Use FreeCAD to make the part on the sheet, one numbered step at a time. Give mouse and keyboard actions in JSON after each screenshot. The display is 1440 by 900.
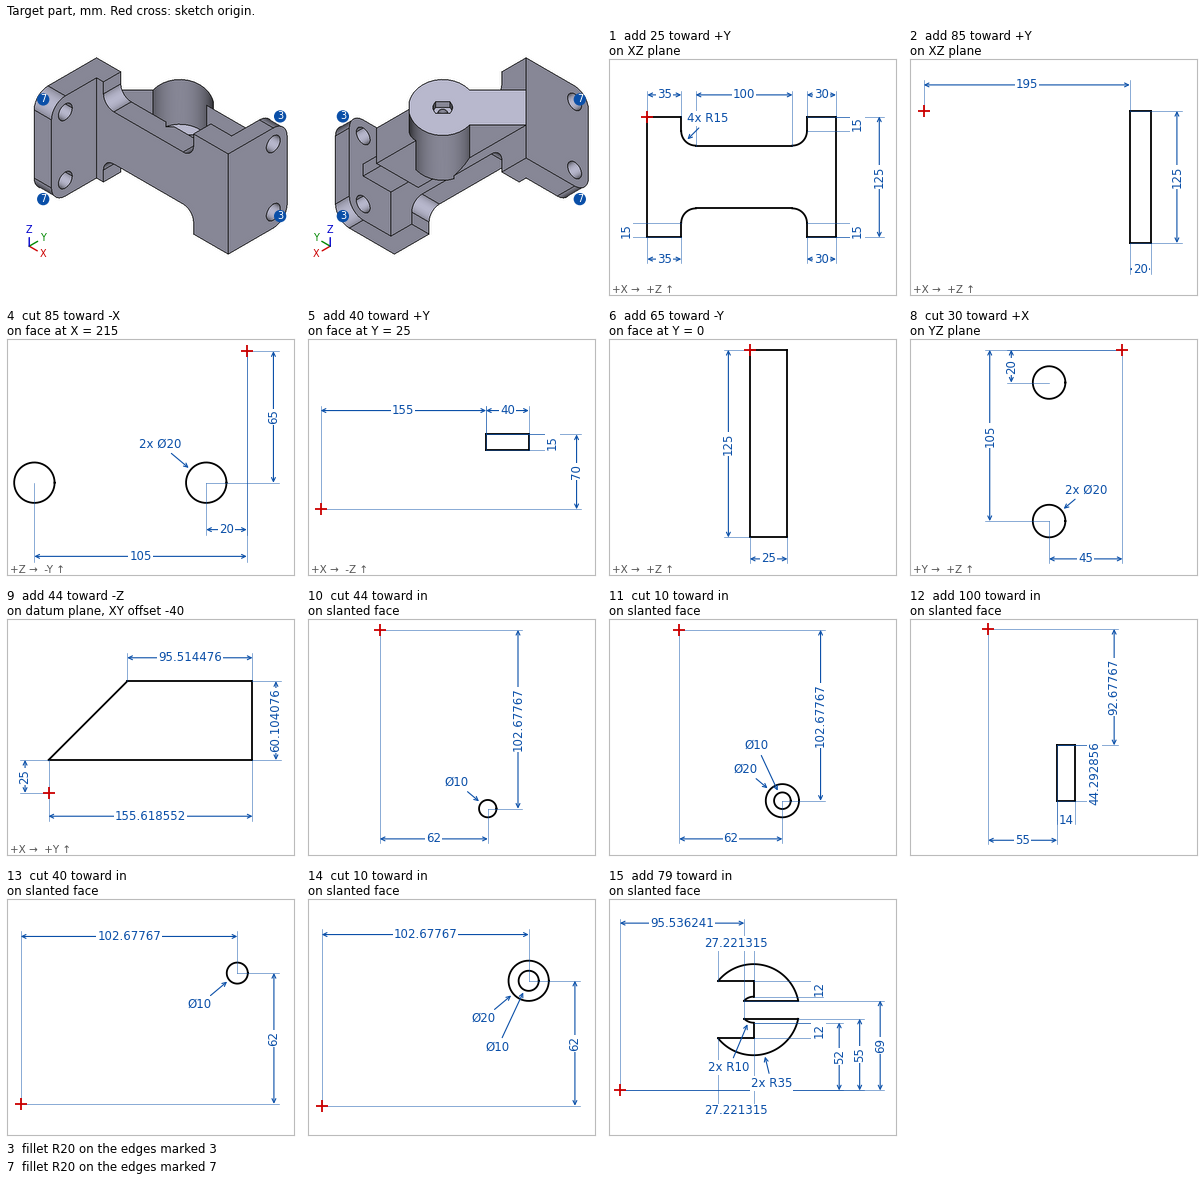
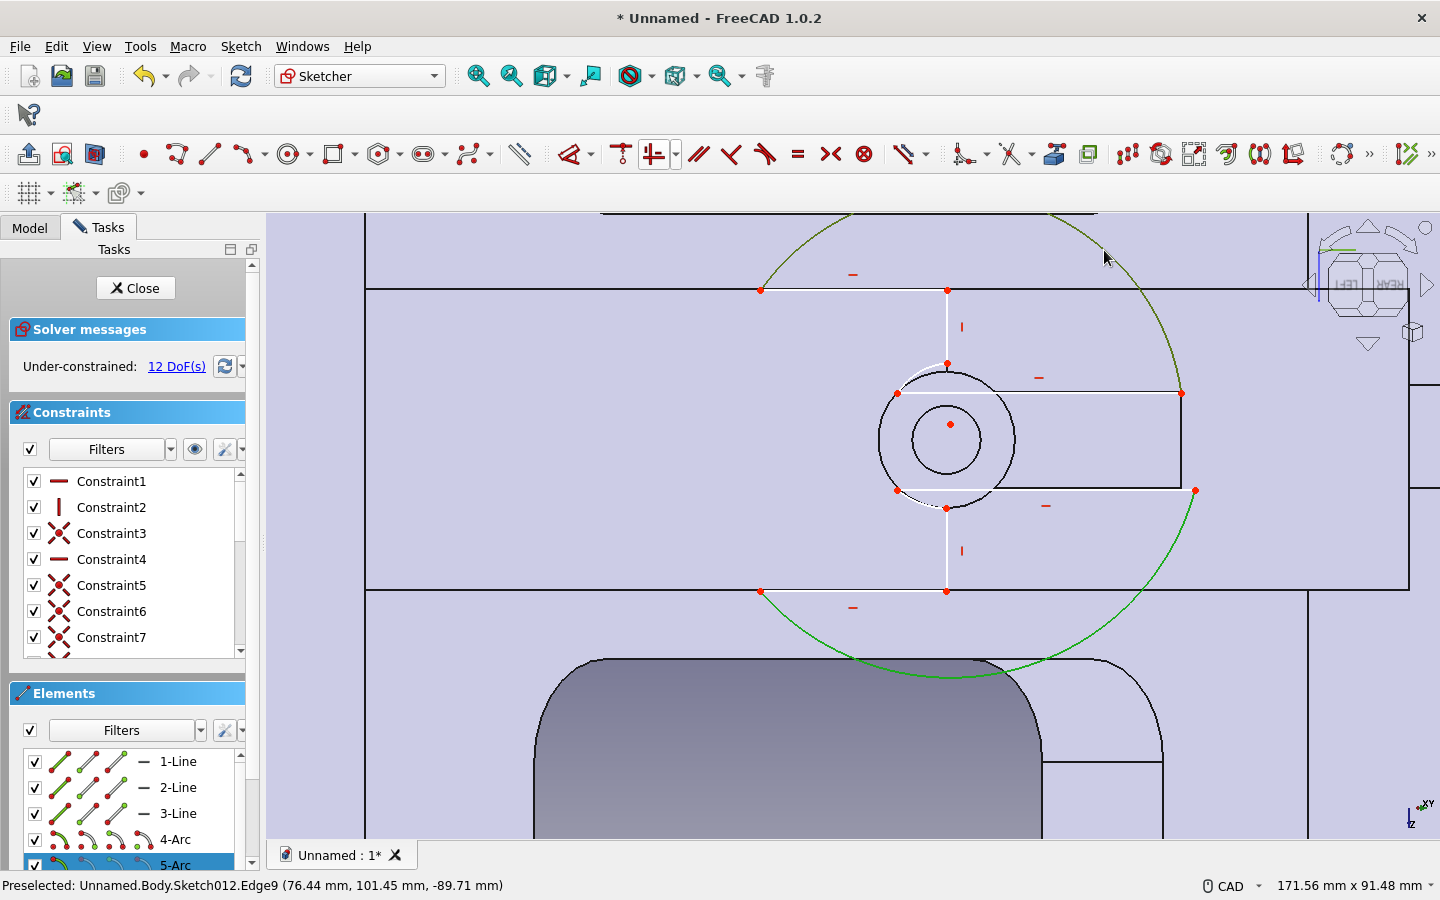
{"action": "left_click", "coordinate": [798, 154]}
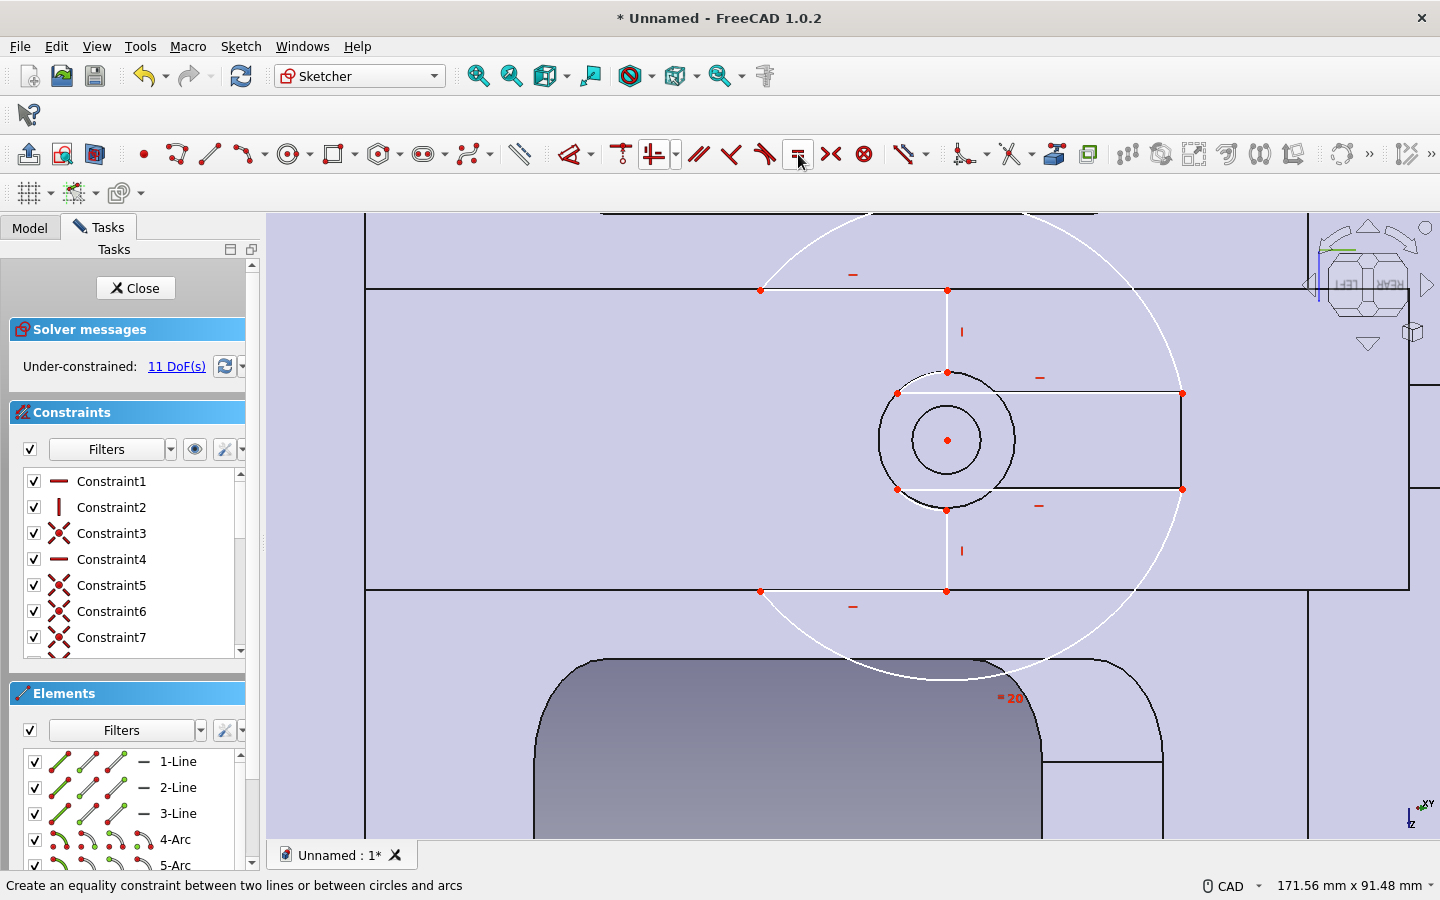
{"action": "scroll", "coordinate": [910, 500], "scroll_direction": "up", "scroll_amount": 2}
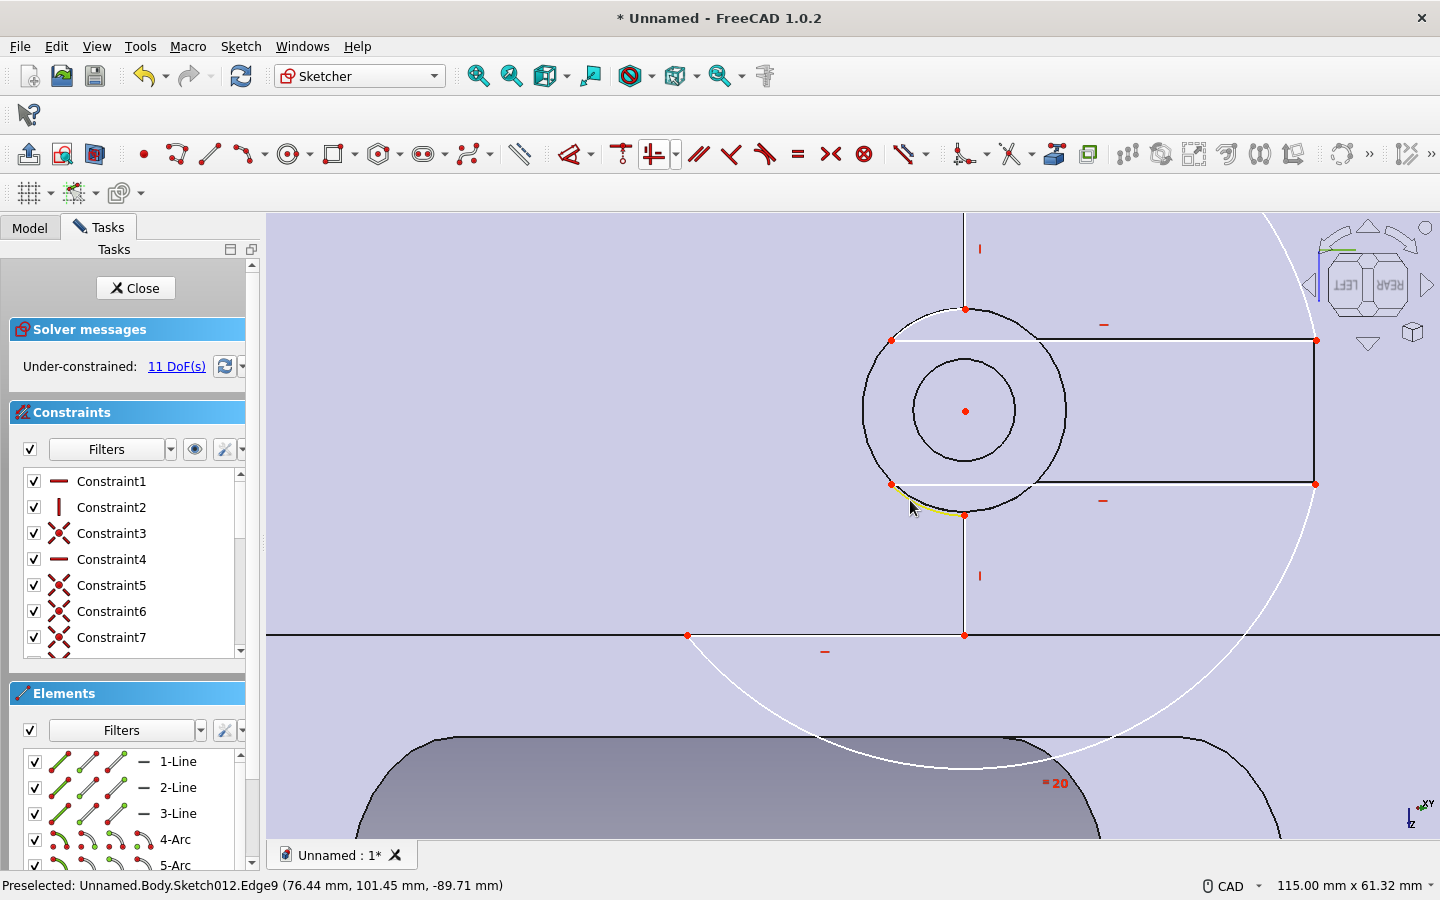
{"action": "left_click", "coordinate": [910, 500]}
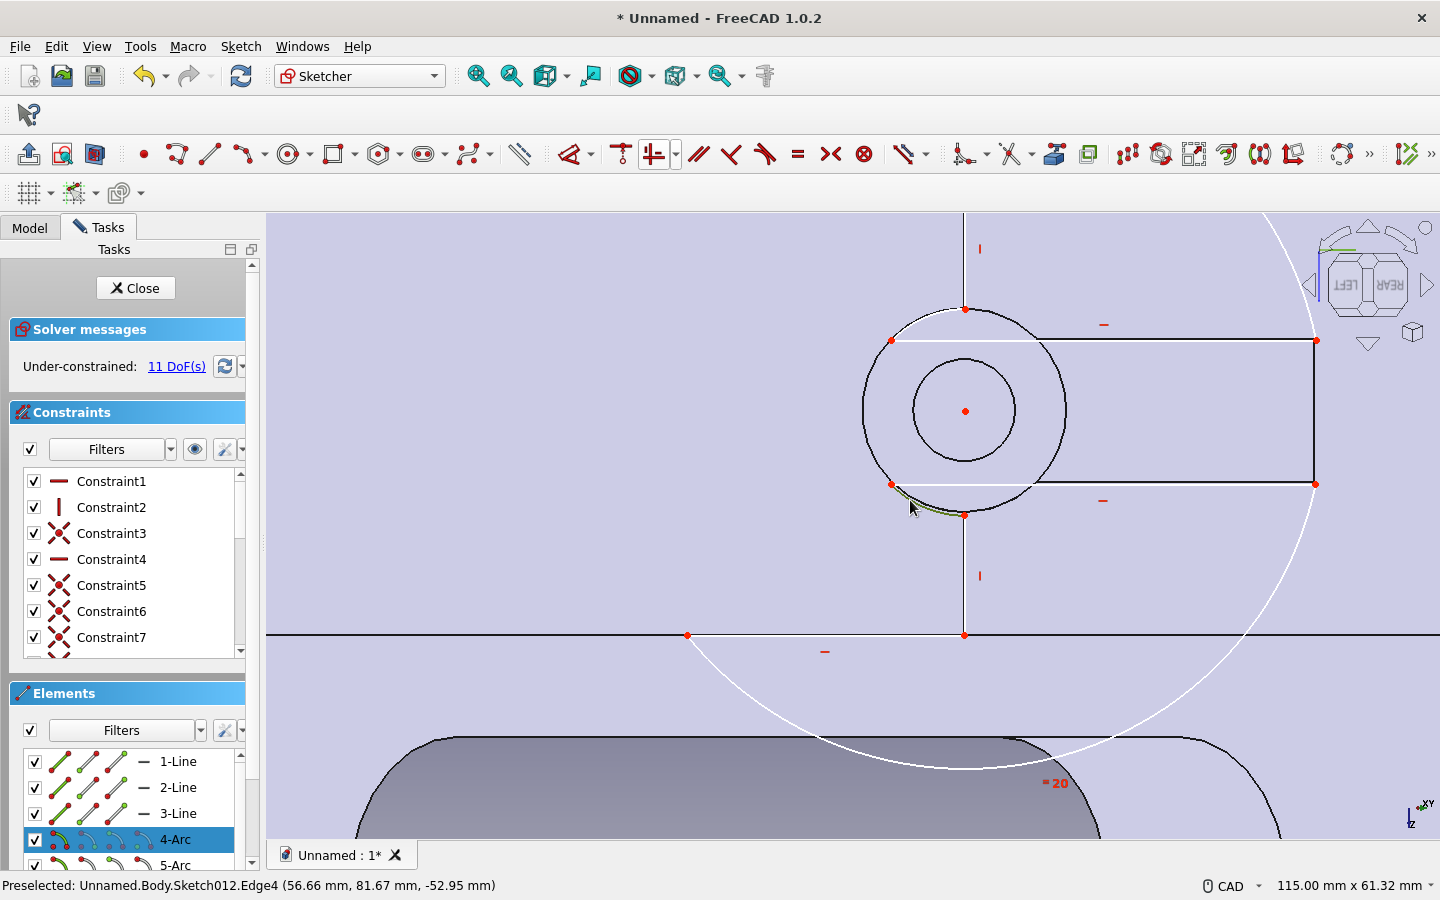
{"action": "left_click", "coordinate": [941, 312]}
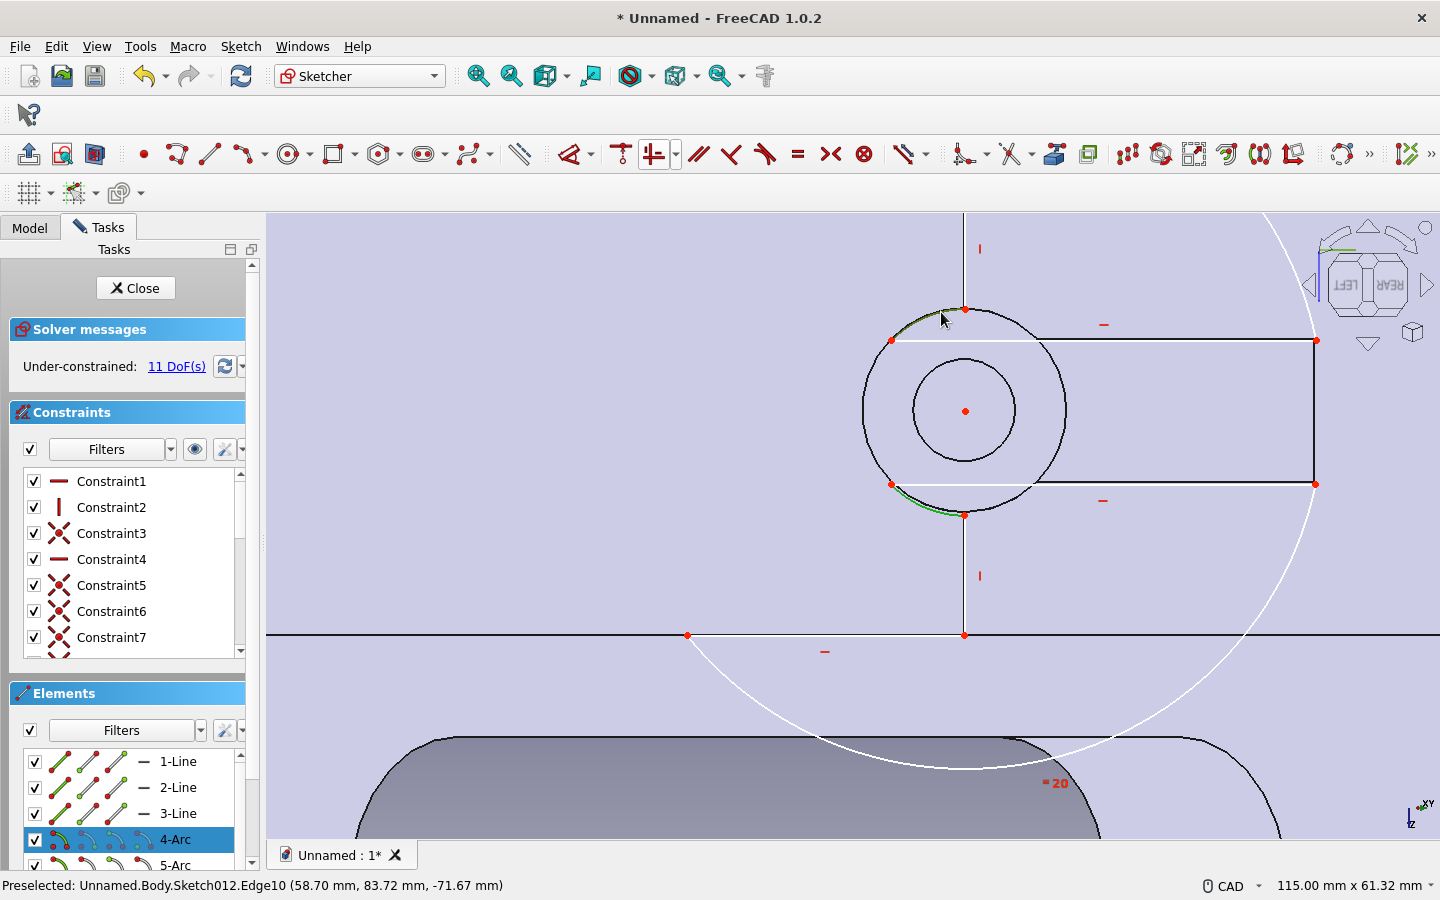
{"action": "key", "text": "e"}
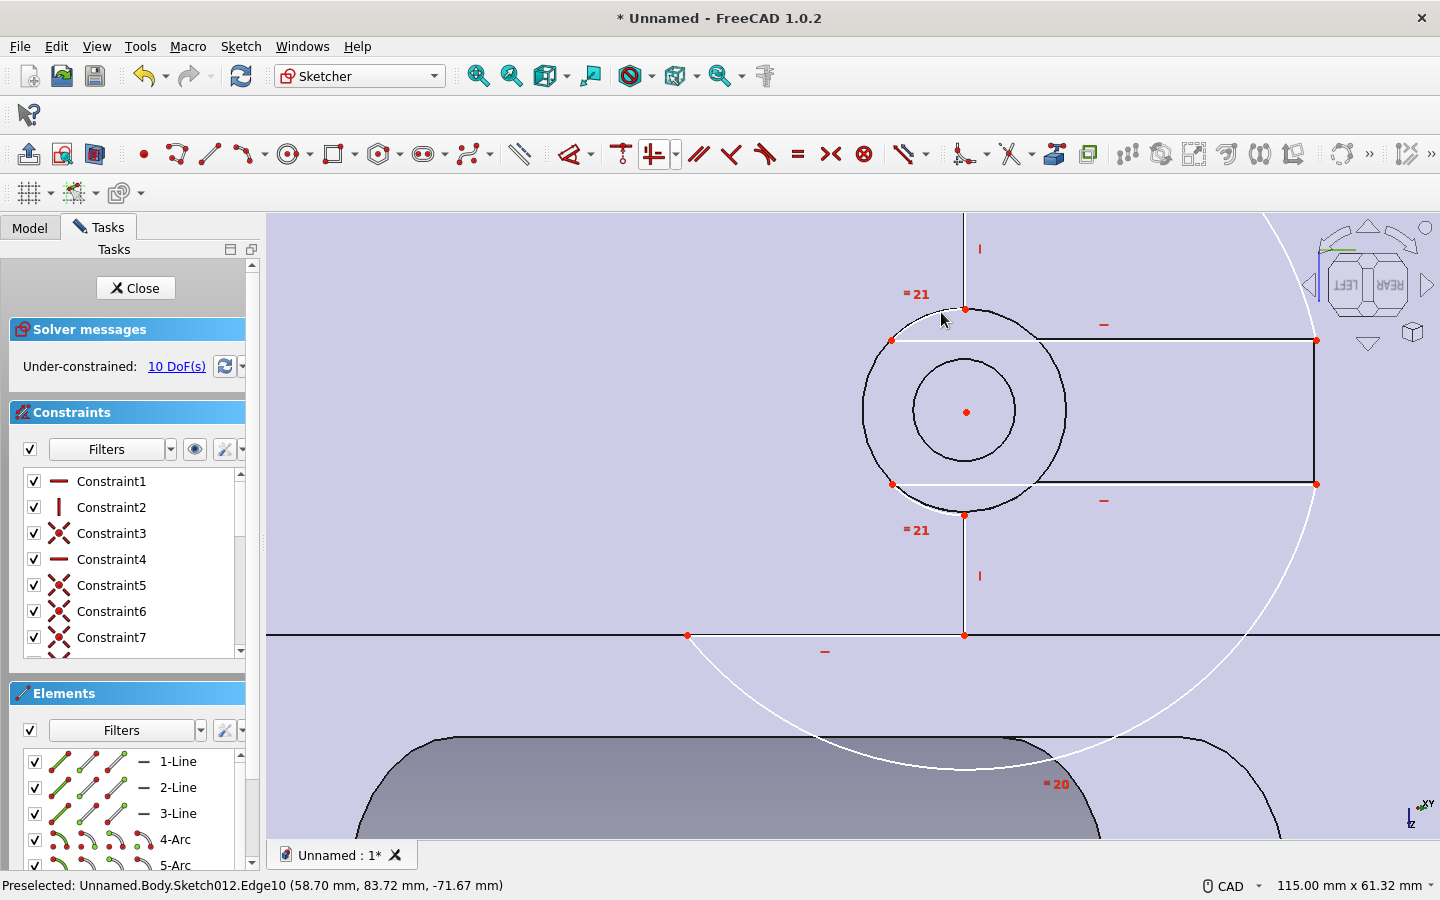
{"action": "left_click", "coordinate": [568, 154]}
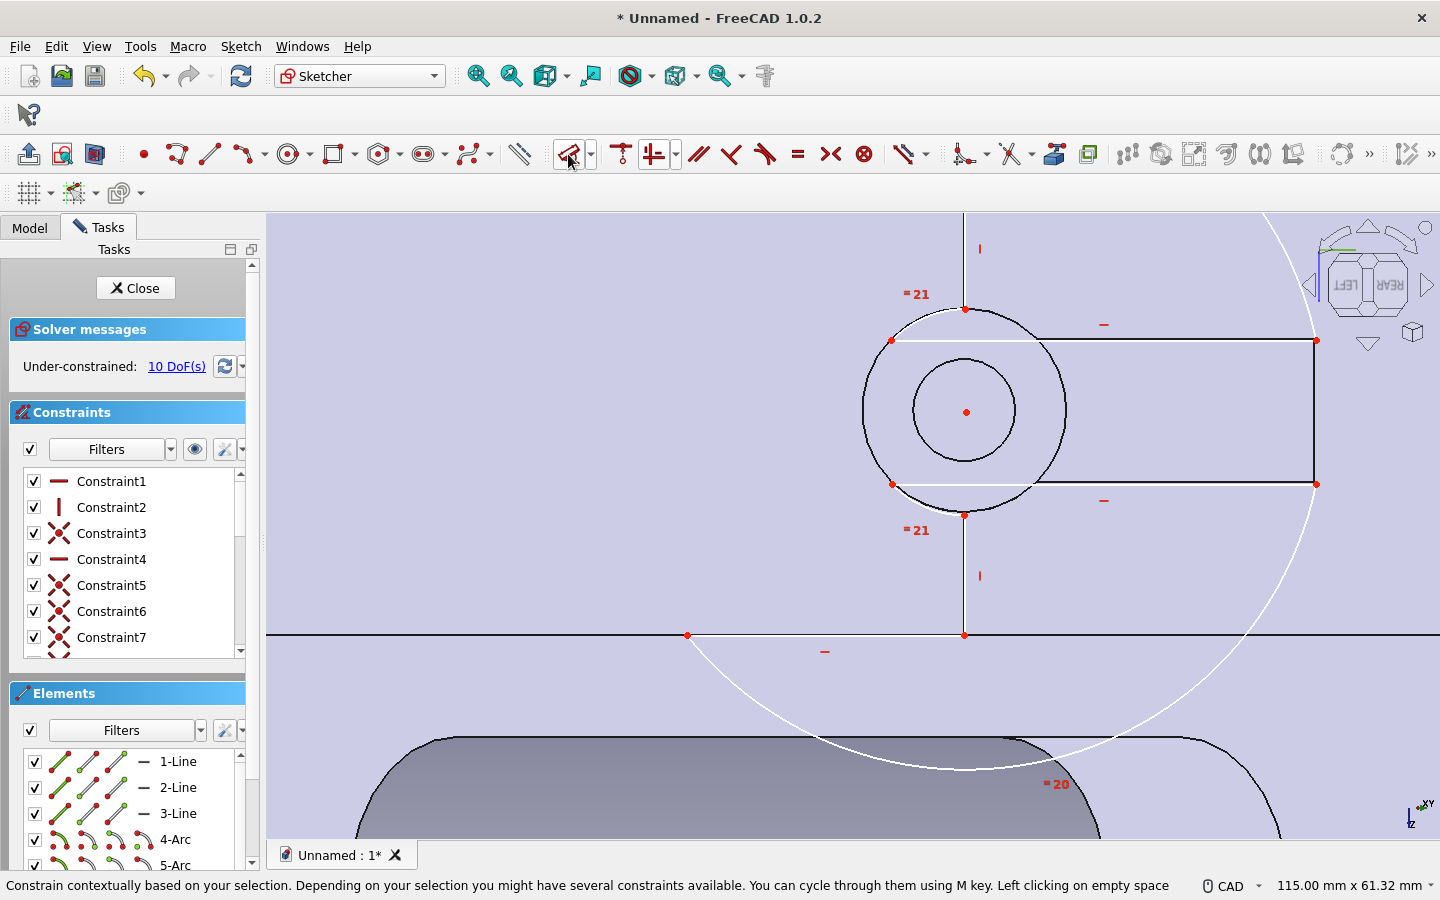
{"action": "left_click", "coordinate": [911, 500]}
{"action": "left_click", "coordinate": [894, 527]}